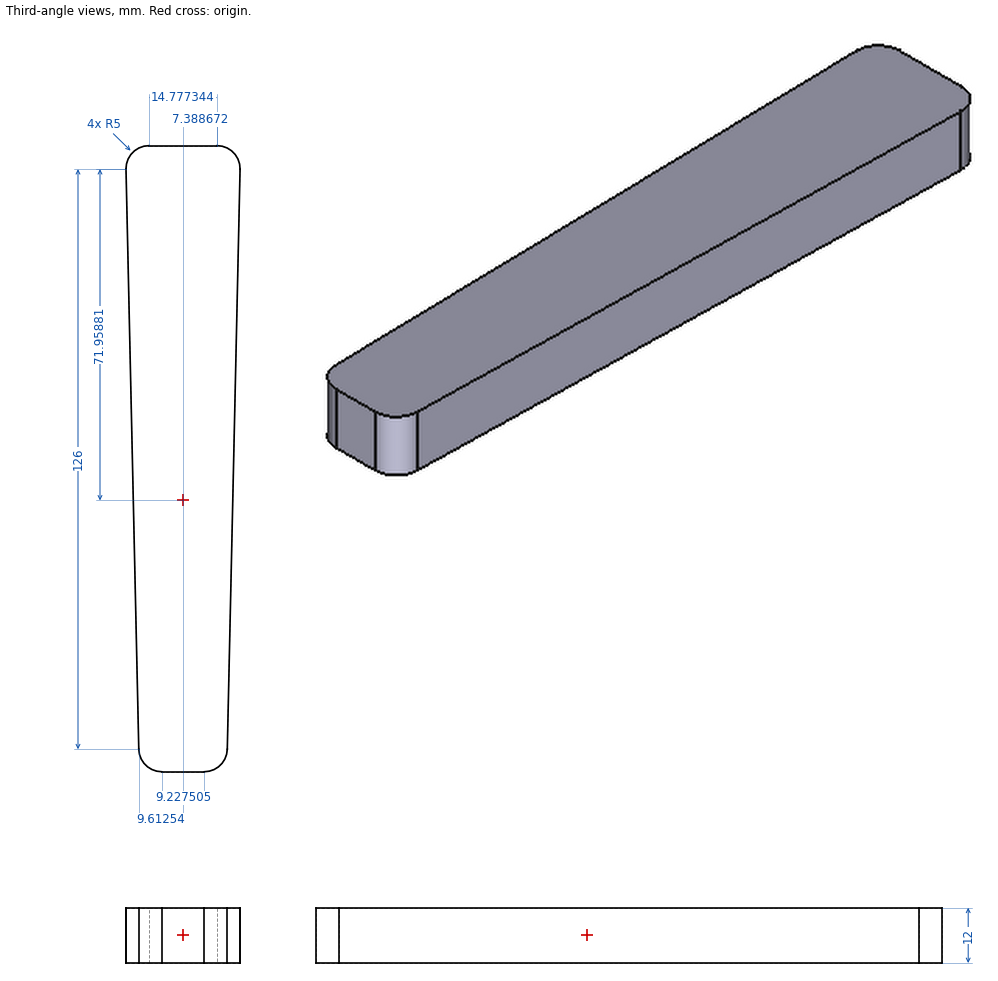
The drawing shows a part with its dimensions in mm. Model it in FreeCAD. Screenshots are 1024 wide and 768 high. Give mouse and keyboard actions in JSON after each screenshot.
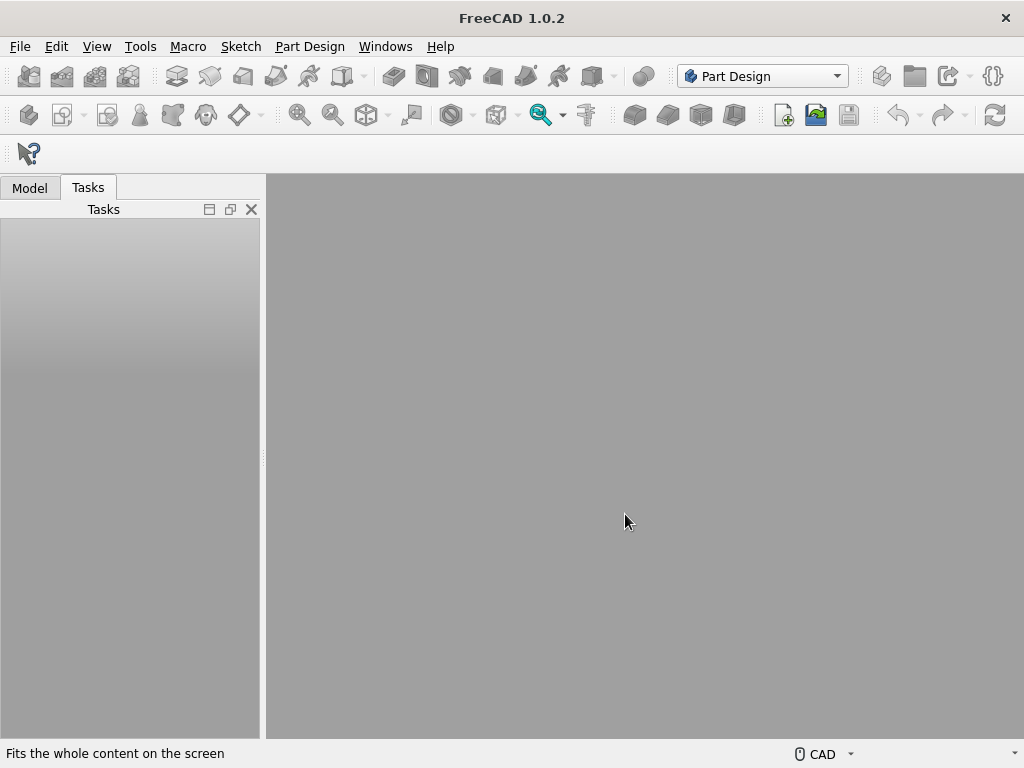
{"action": "key", "text": "ctrl+n"}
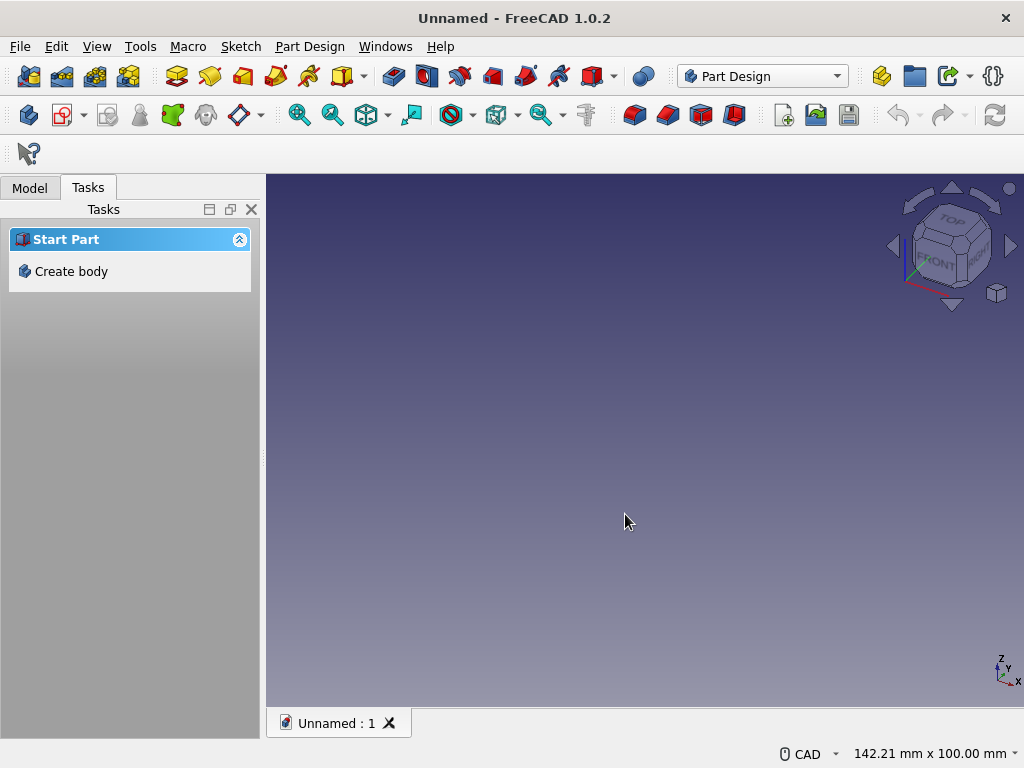
{"action": "left_click", "coordinate": [62, 116]}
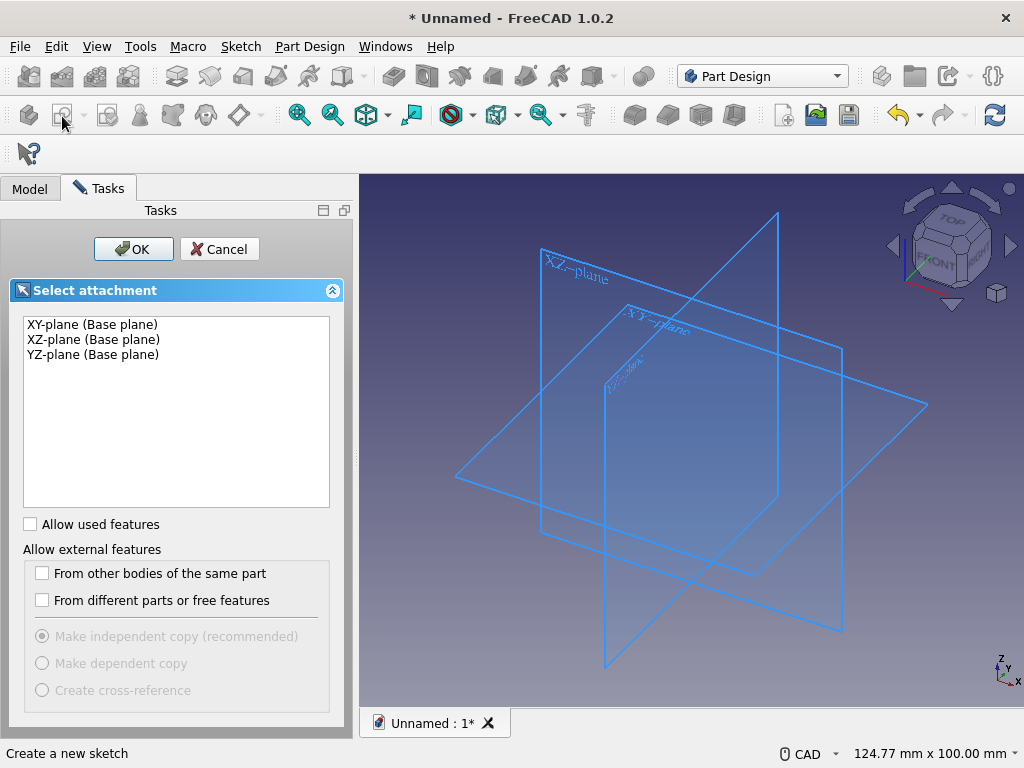
{"action": "left_click", "coordinate": [84, 324]}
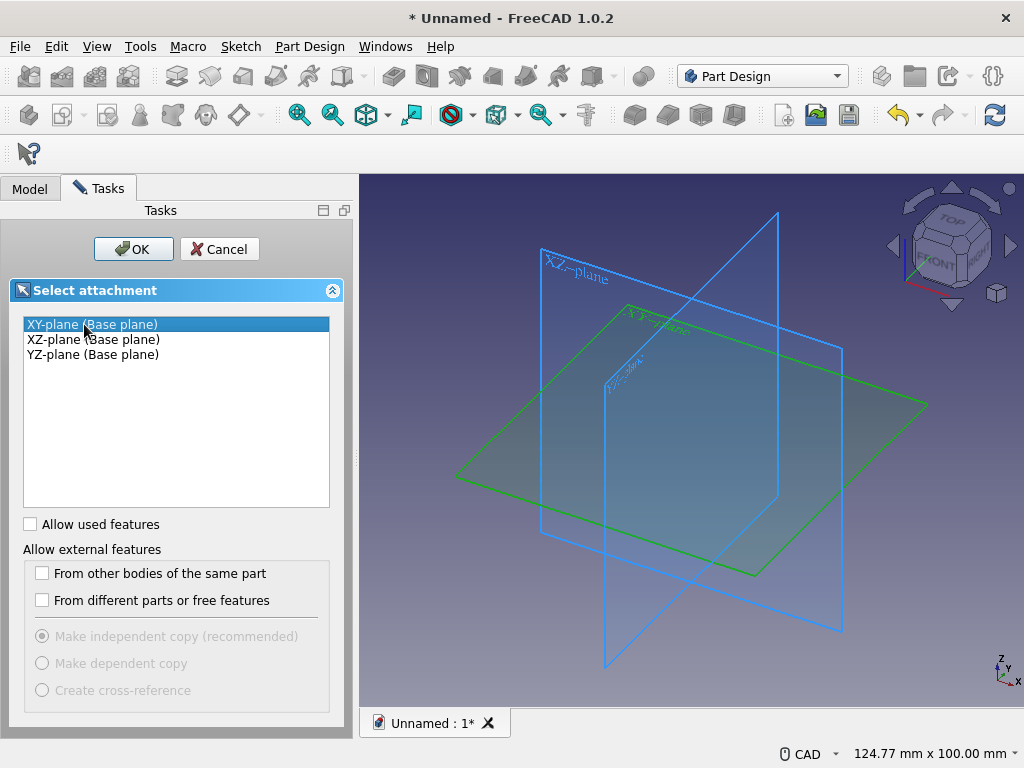
{"action": "left_click", "coordinate": [134, 249]}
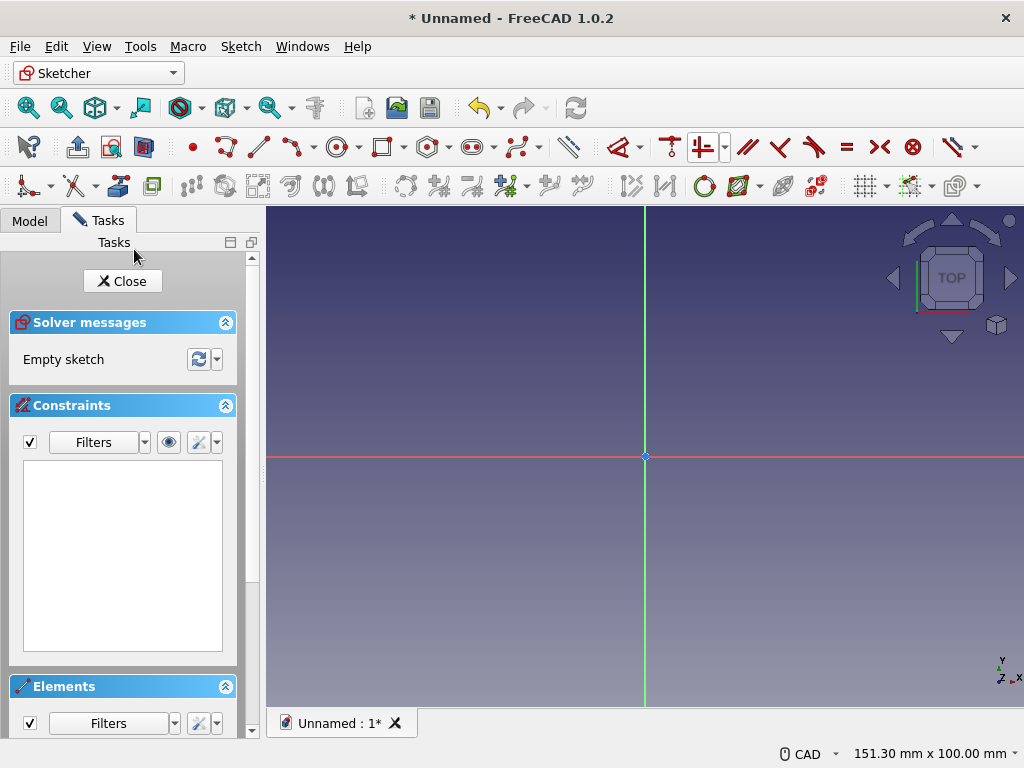
{"action": "scroll", "coordinate": [521, 494], "scroll_direction": "down", "scroll_amount": 4}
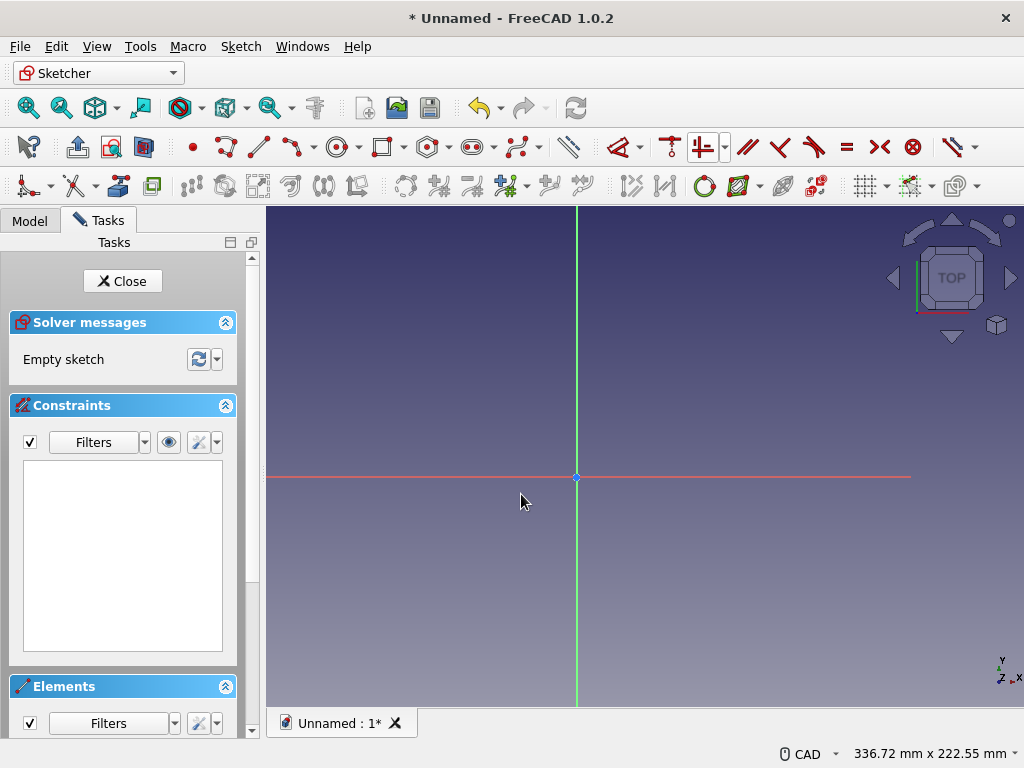
{"action": "key", "text": "g l"}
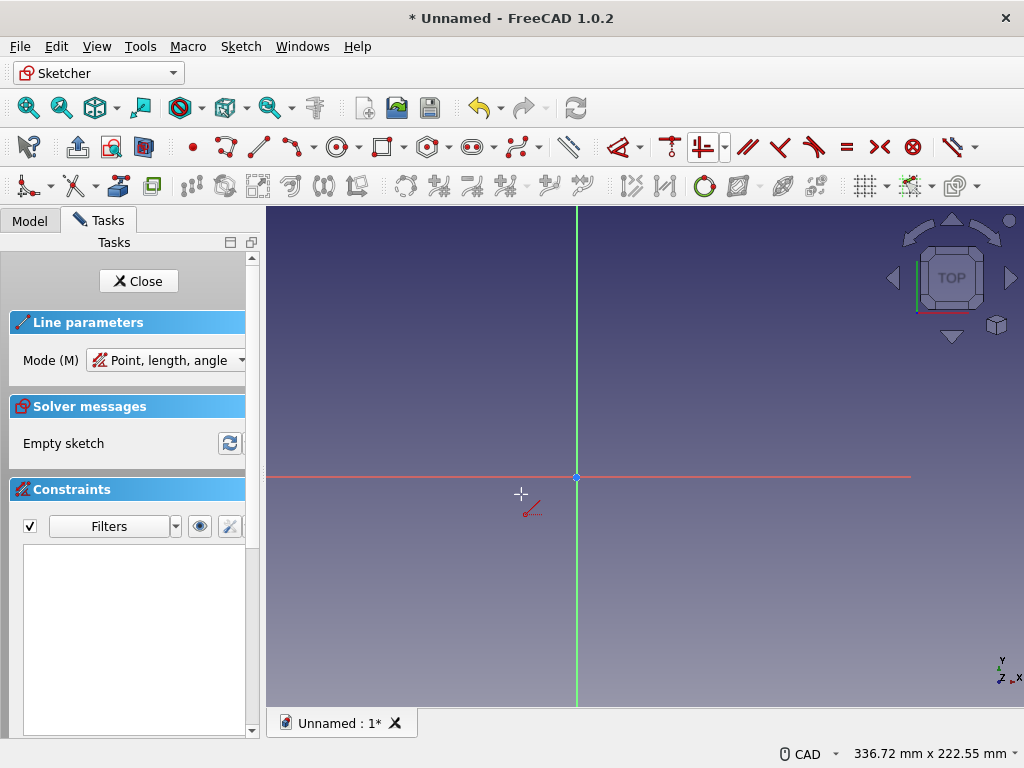
{"action": "left_click", "coordinate": [594, 304]}
{"action": "left_click", "coordinate": [560, 304]}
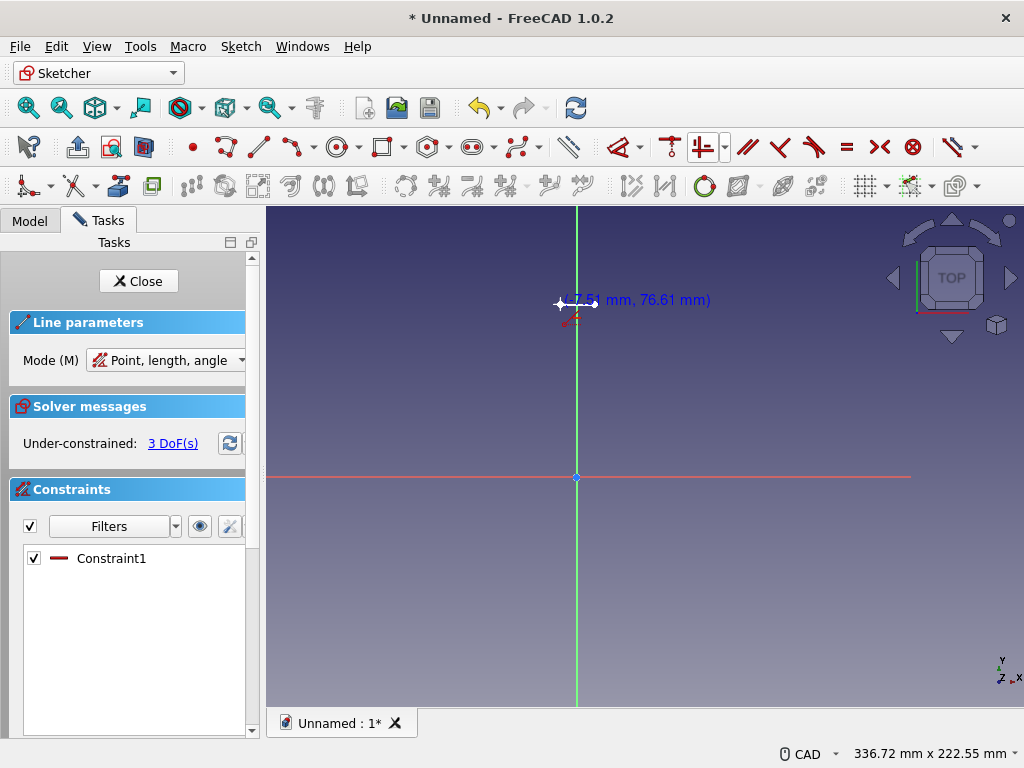
{"action": "left_click", "coordinate": [549, 315]}
{"action": "left_click", "coordinate": [563, 599]}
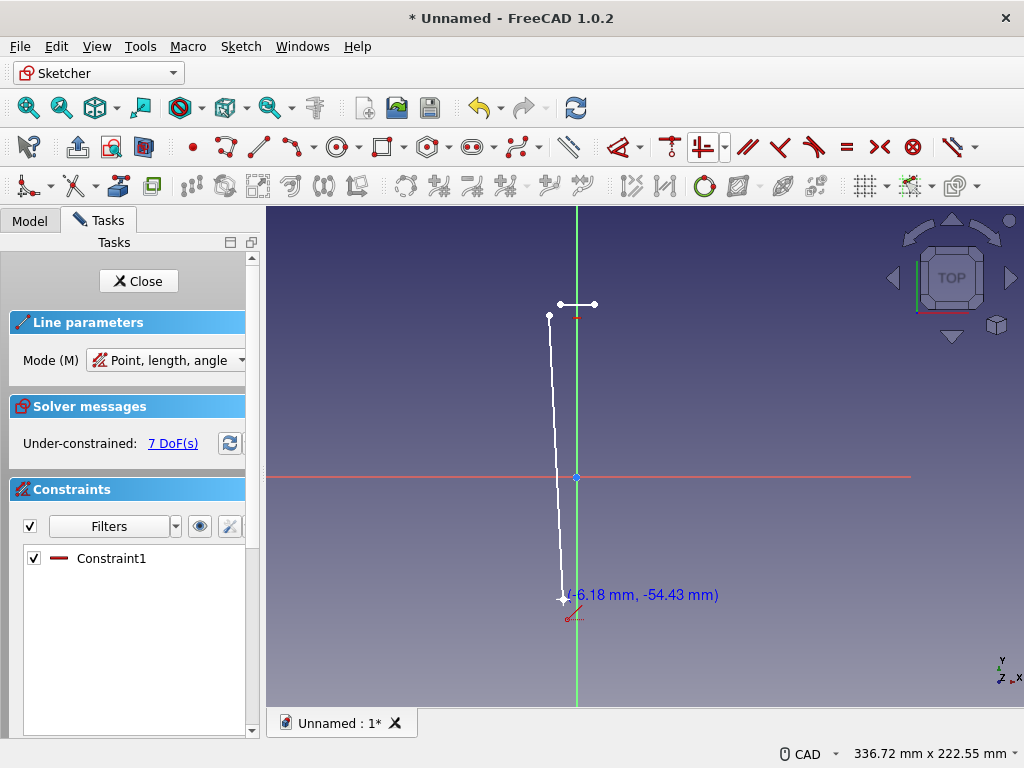
{"action": "scroll", "coordinate": [567, 610], "scroll_direction": "up", "scroll_amount": 3}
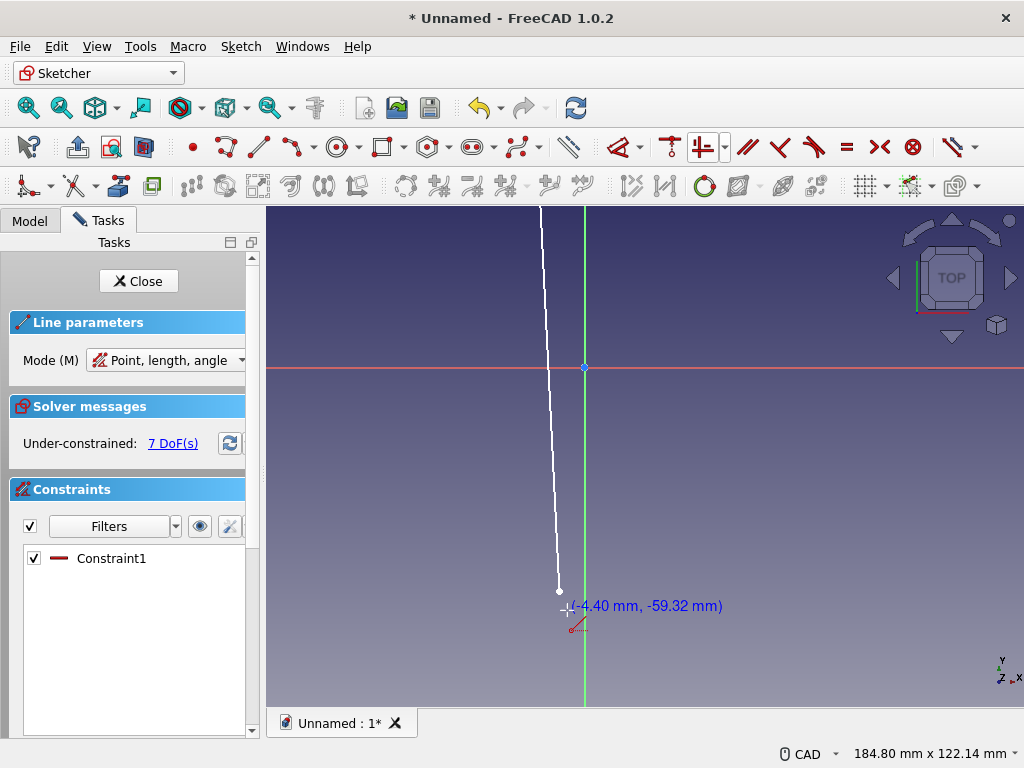
{"action": "left_click", "coordinate": [566, 610]}
{"action": "left_click", "coordinate": [604, 610]}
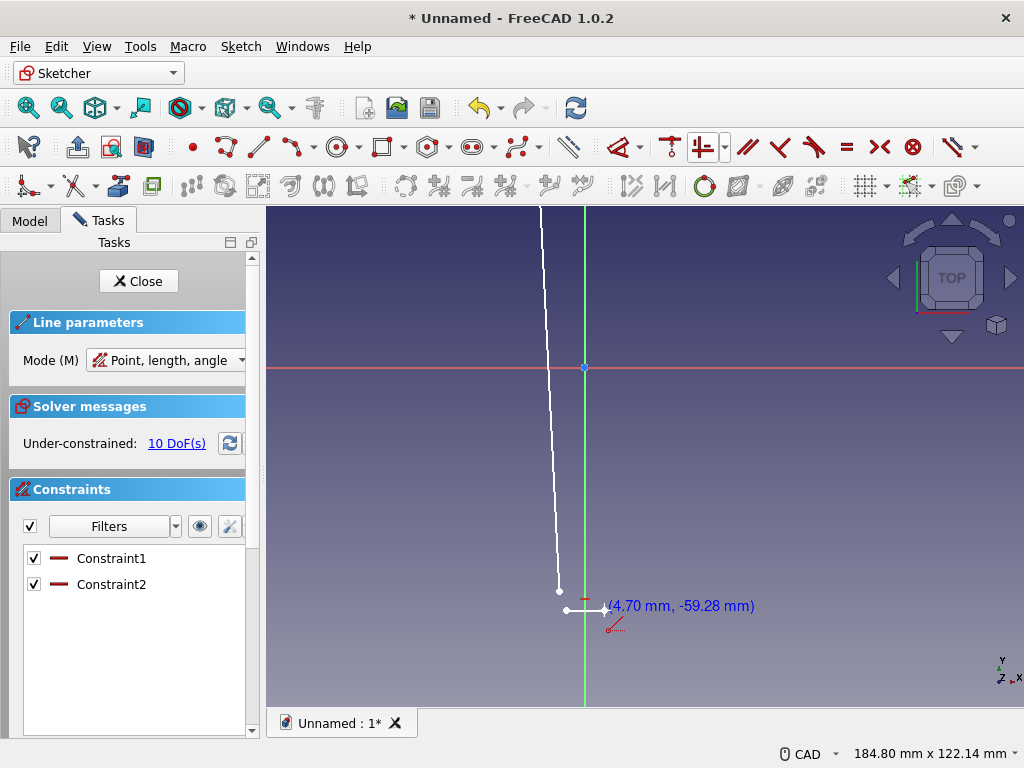
{"action": "left_click", "coordinate": [624, 590]}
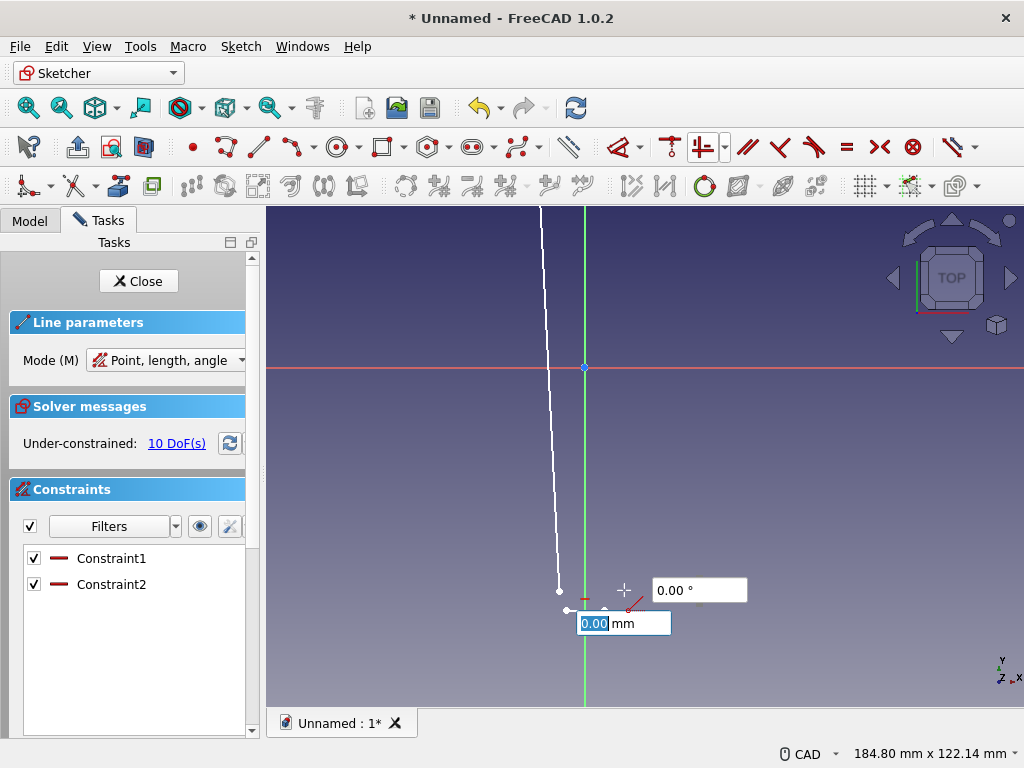
{"action": "scroll", "coordinate": [567, 610], "scroll_direction": "down", "scroll_amount": 3}